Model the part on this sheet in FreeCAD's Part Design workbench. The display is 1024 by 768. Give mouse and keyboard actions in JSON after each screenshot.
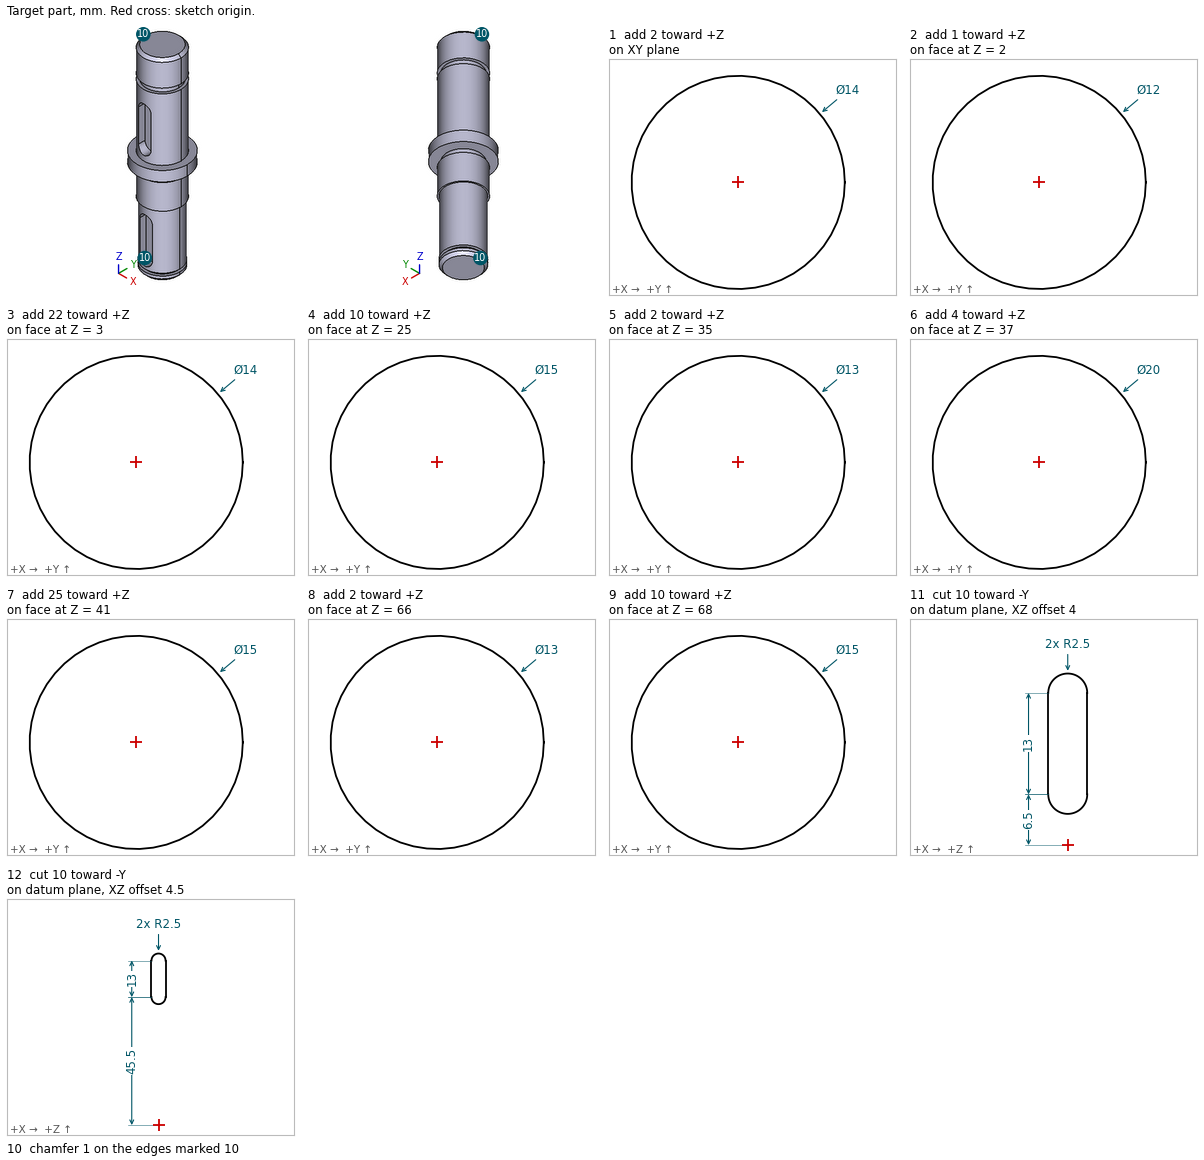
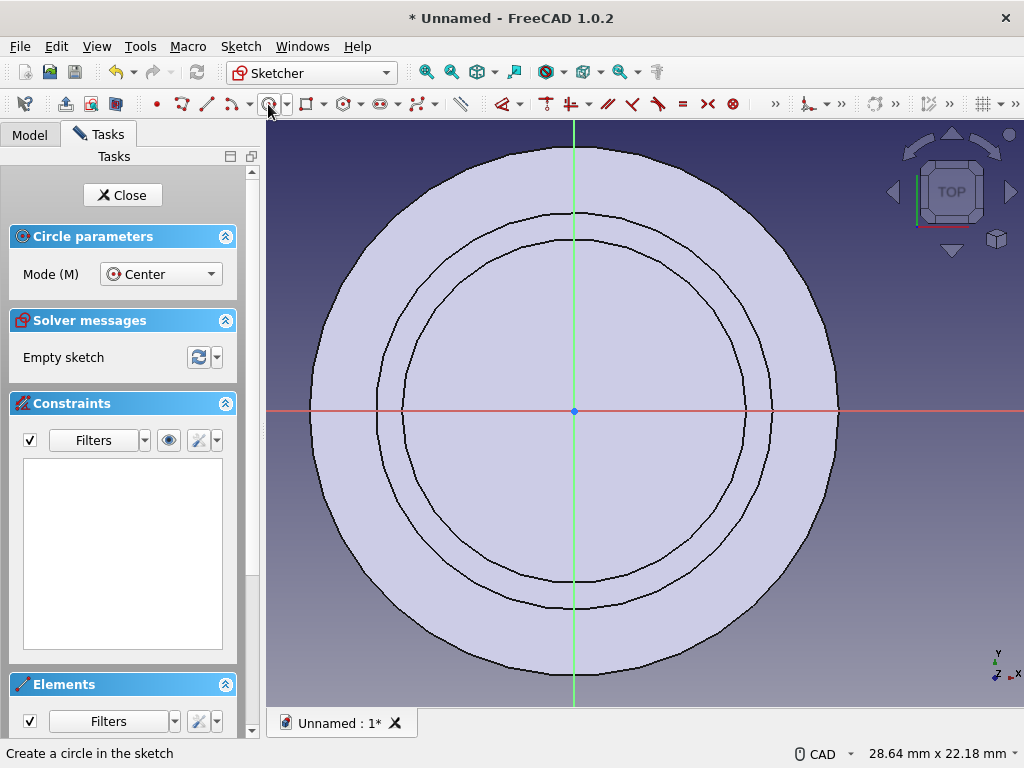
{"action": "left_click", "coordinate": [574, 411]}
{"action": "left_click", "coordinate": [715, 271]}
{"action": "key", "text": "Escape"}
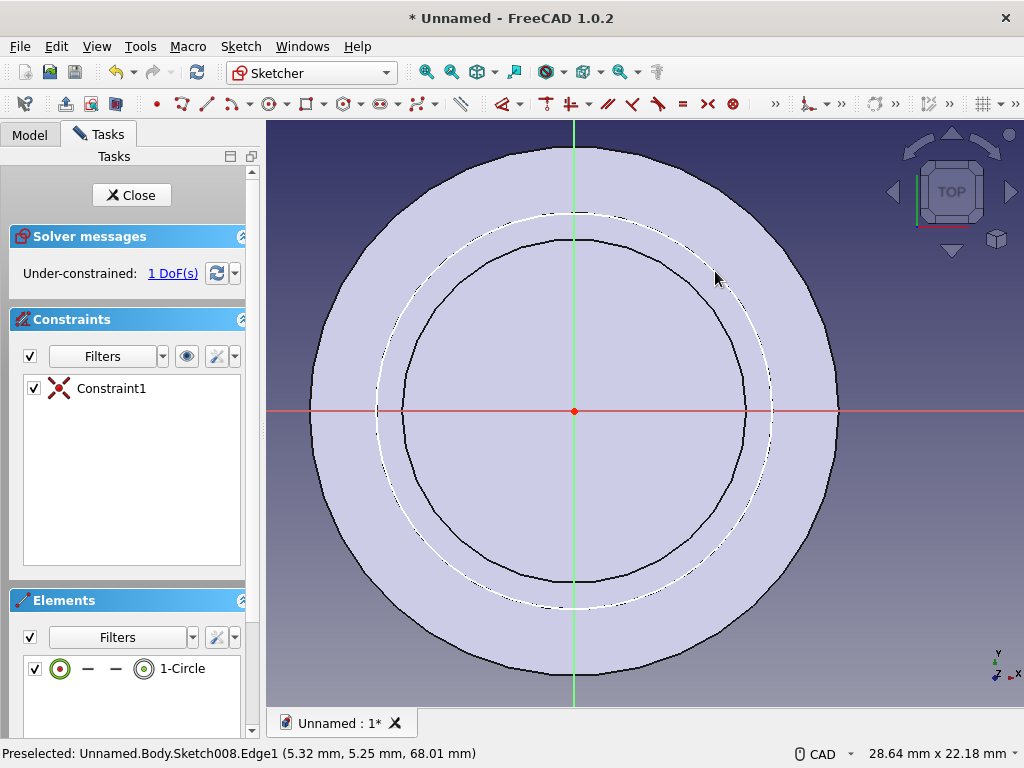
{"action": "key", "text": "d"}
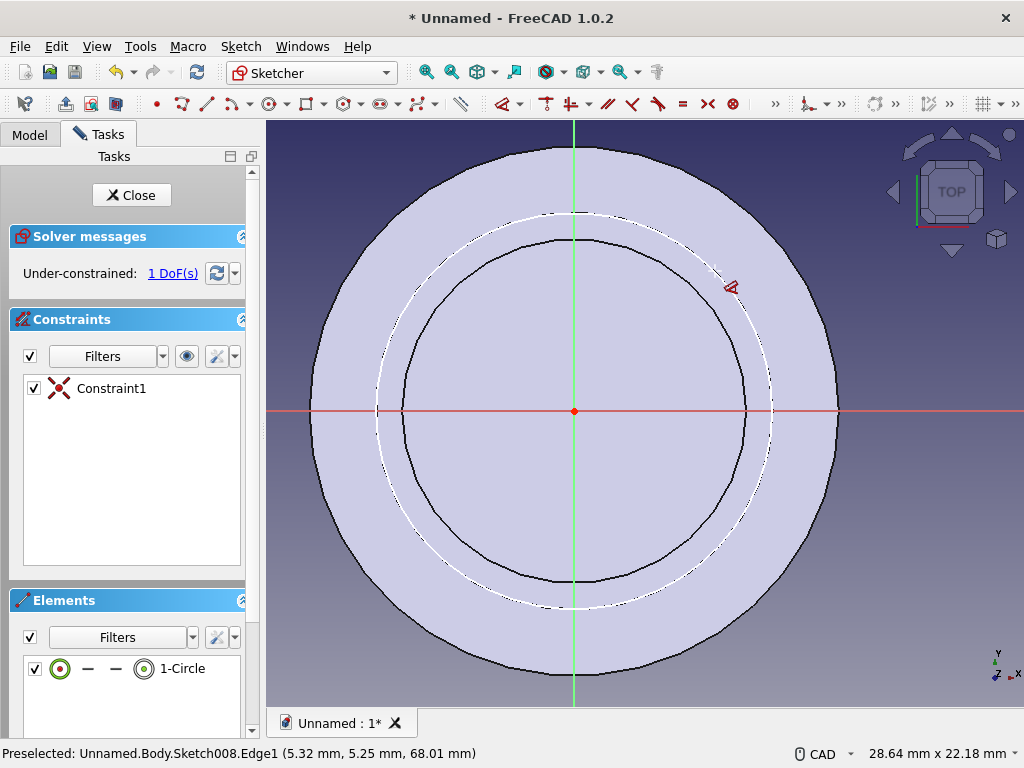
{"action": "left_click", "coordinate": [714, 271]}
{"action": "left_click", "coordinate": [737, 248]}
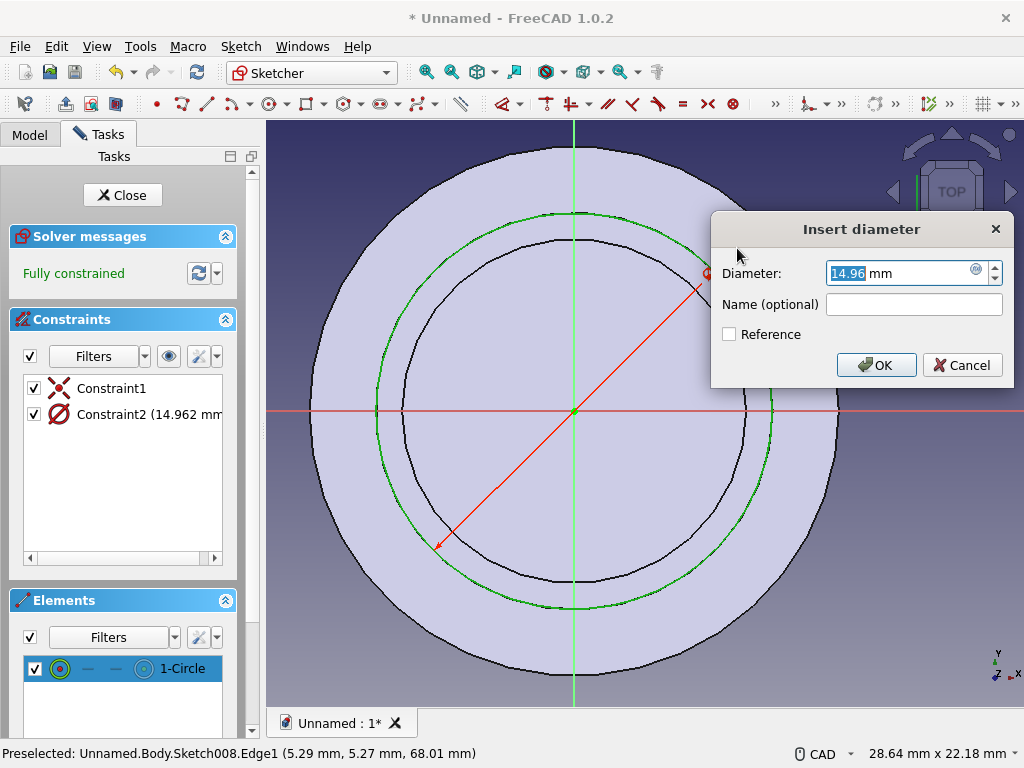
{"action": "type", "text": "15"}
{"action": "key", "text": "Return"}
{"action": "key", "text": "Escape"}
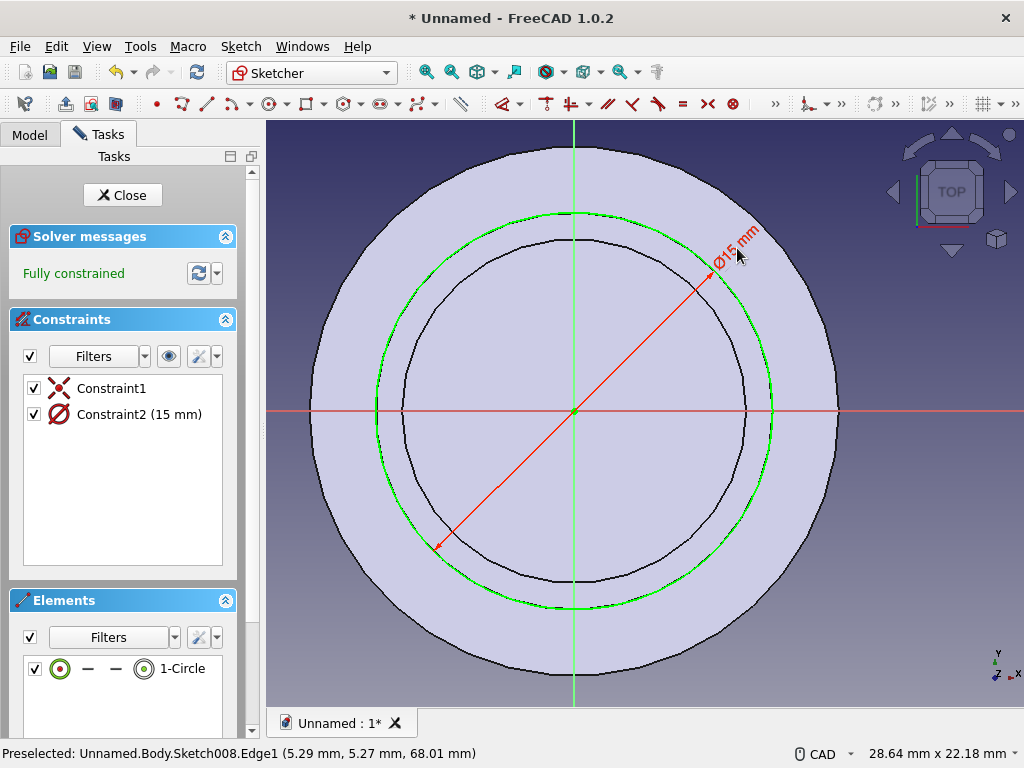
{"action": "left_click", "coordinate": [123, 195]}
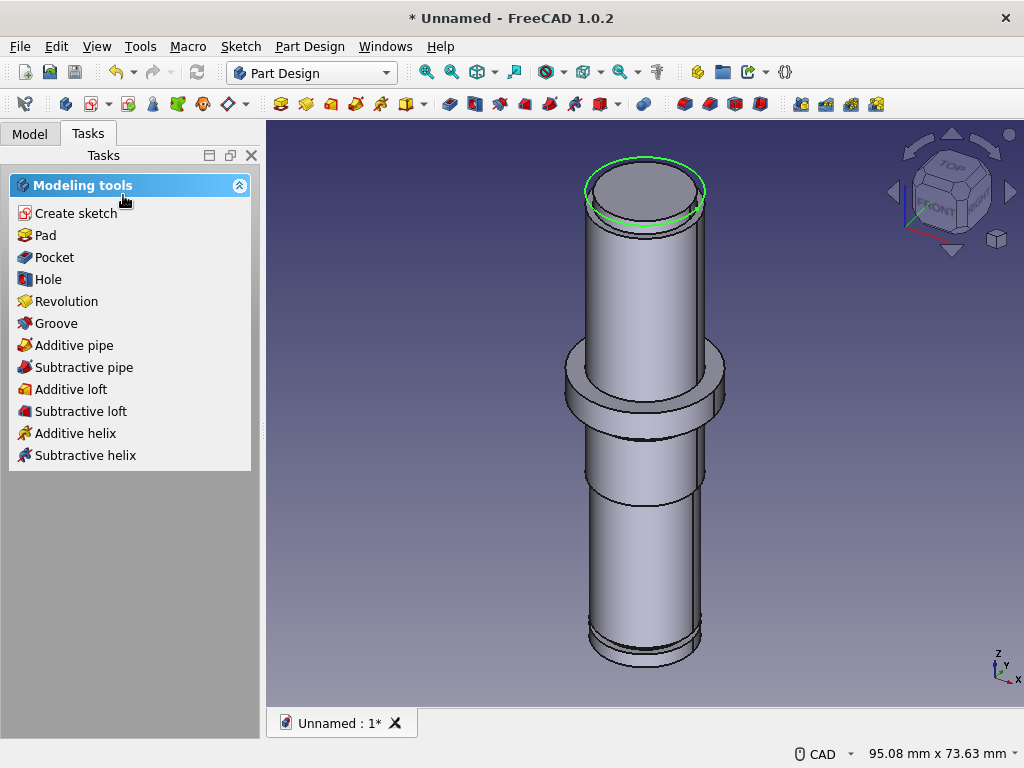
{"action": "left_click", "coordinate": [281, 104]}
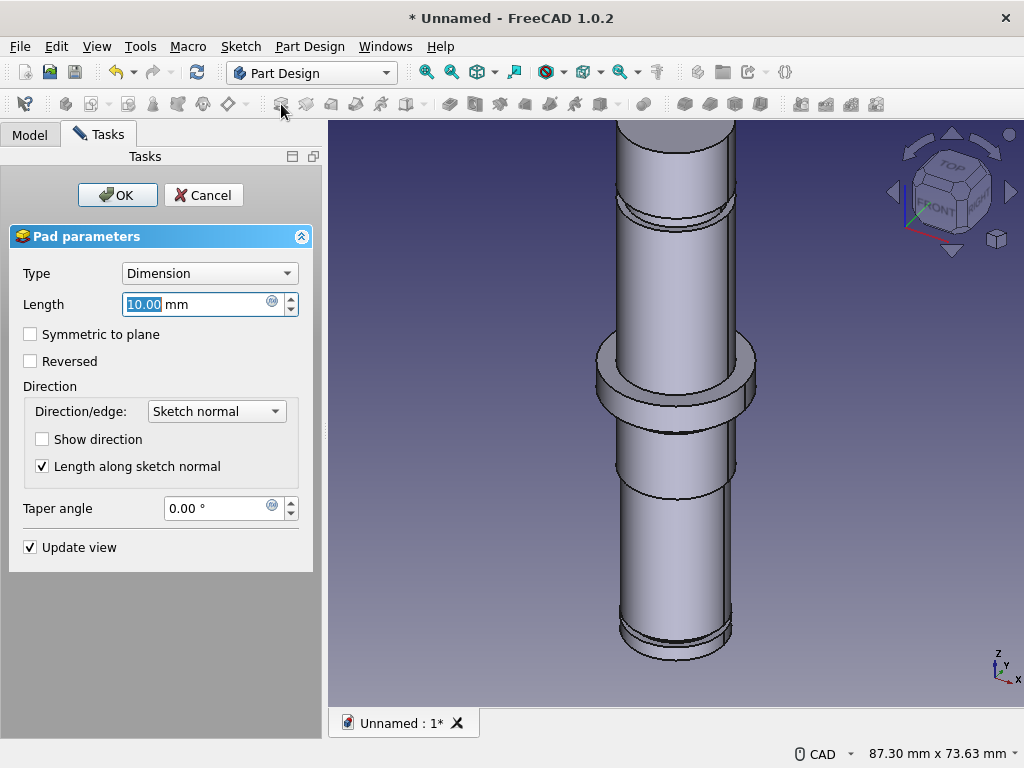
{"action": "type", "text": "10"}
{"action": "key", "text": "Tab"}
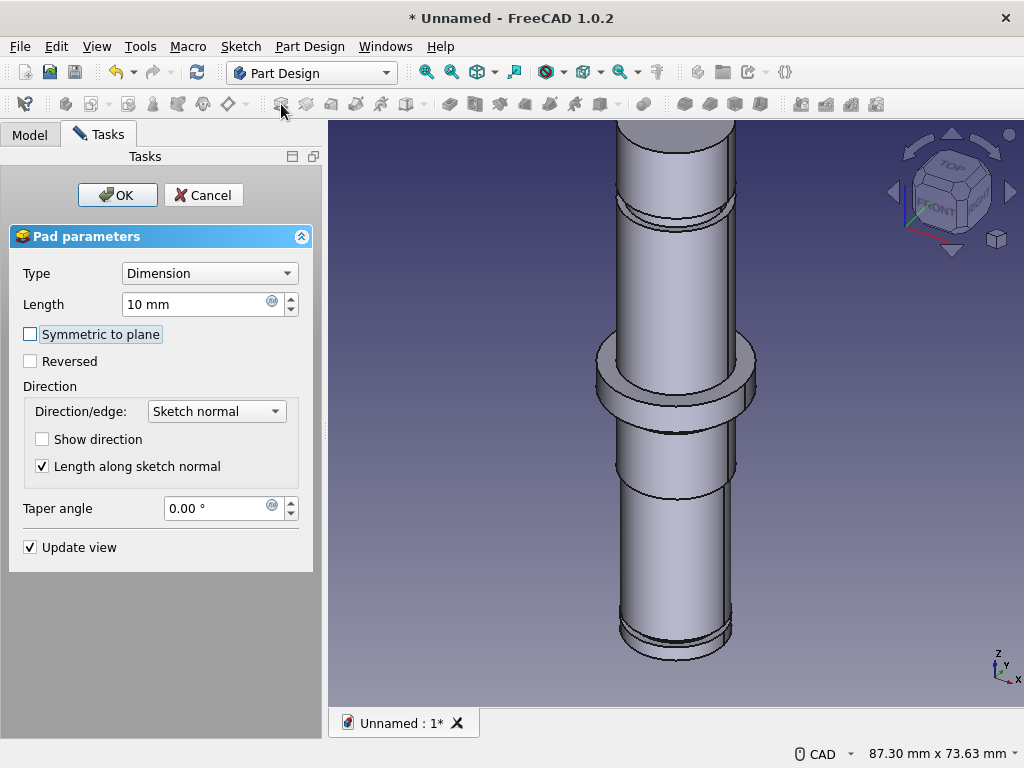
{"action": "left_click", "coordinate": [118, 195]}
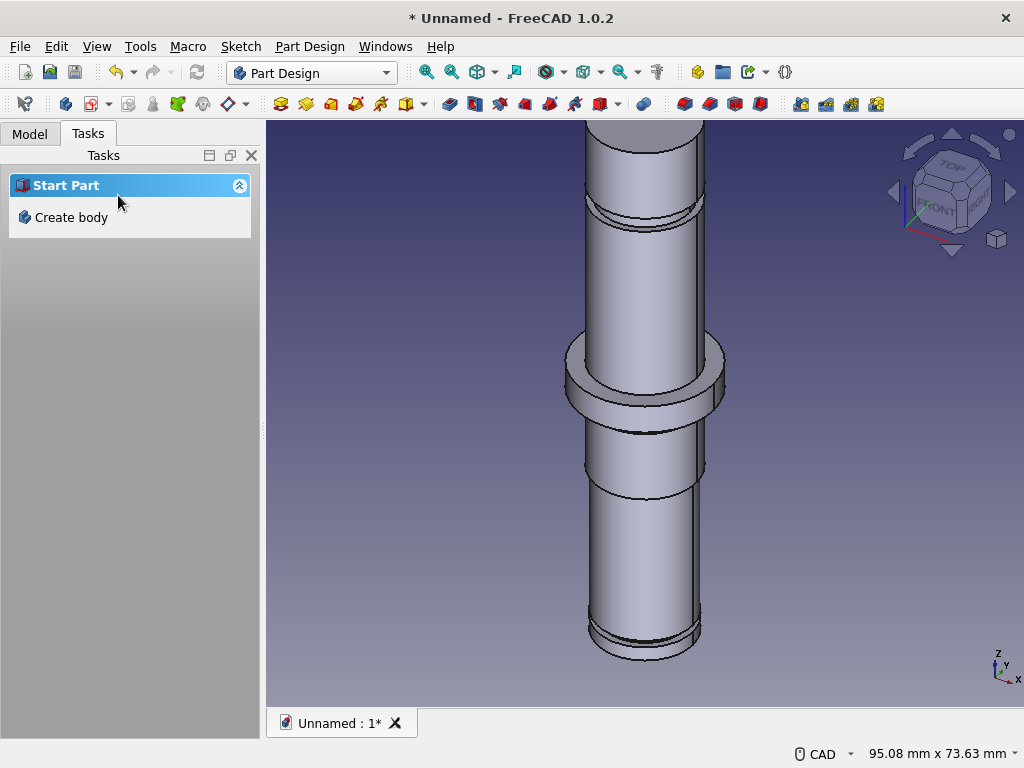
{"action": "left_click", "coordinate": [427, 72]}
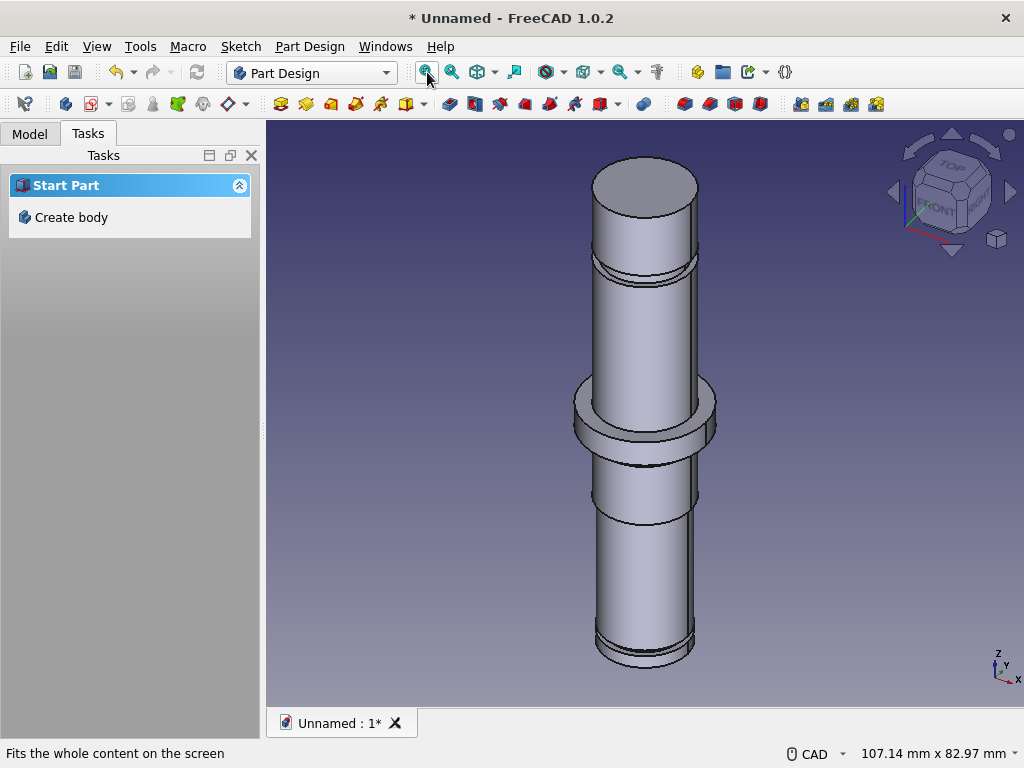
{"action": "left_click", "coordinate": [659, 666]}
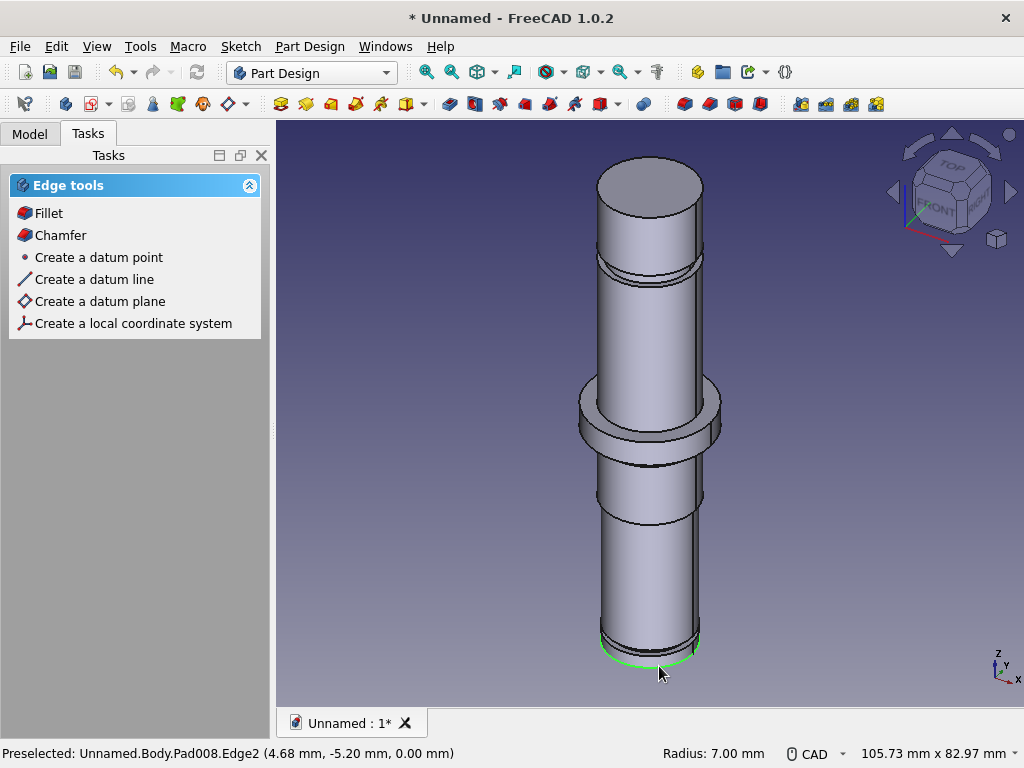
{"action": "left_click", "coordinate": [597, 190], "text": "ctrl"}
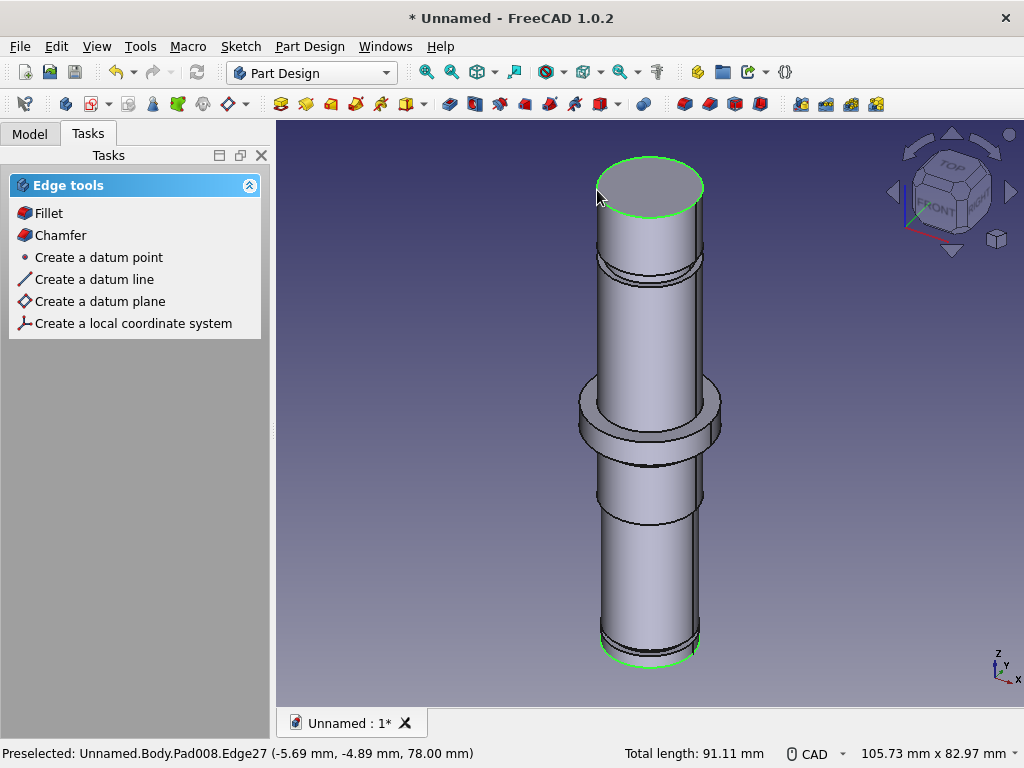
{"action": "left_click", "coordinate": [710, 104]}